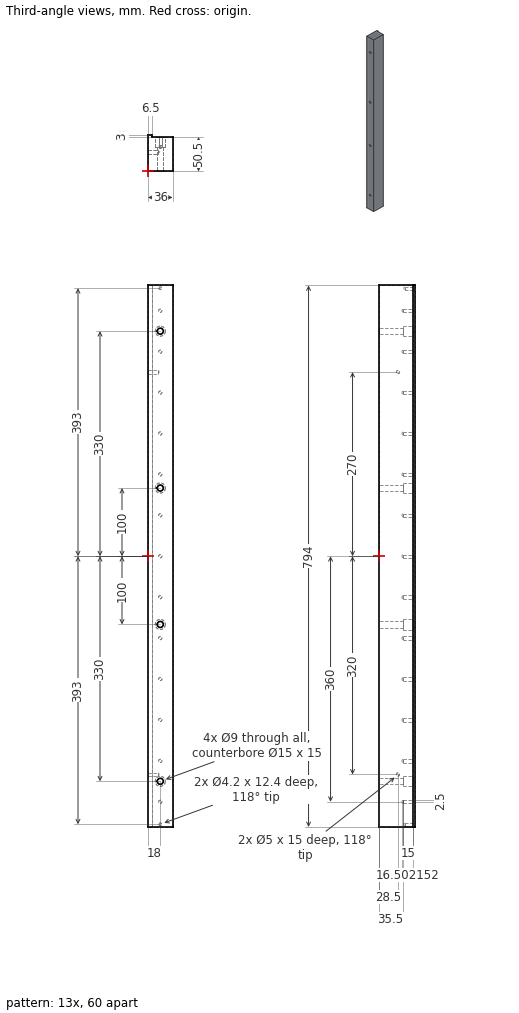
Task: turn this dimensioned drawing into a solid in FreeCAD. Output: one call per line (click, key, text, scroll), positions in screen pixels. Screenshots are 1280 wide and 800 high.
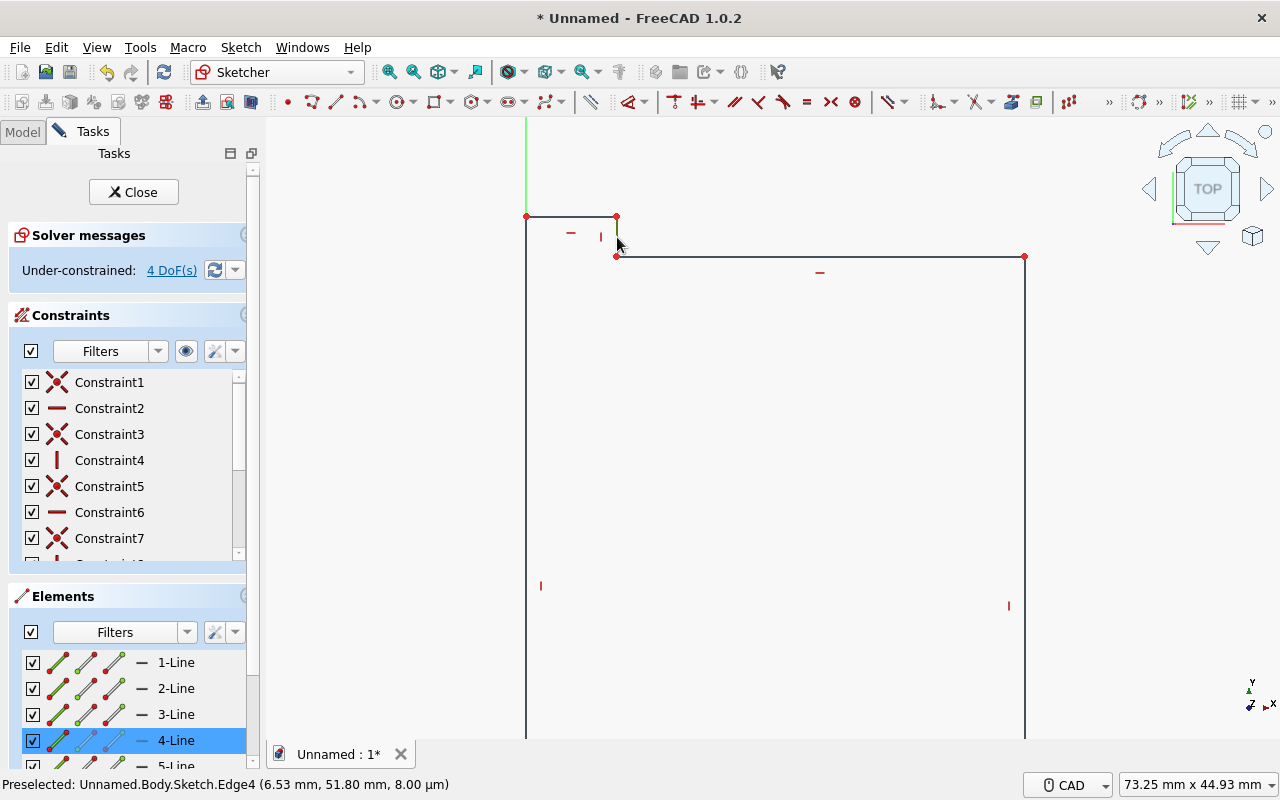
key(i)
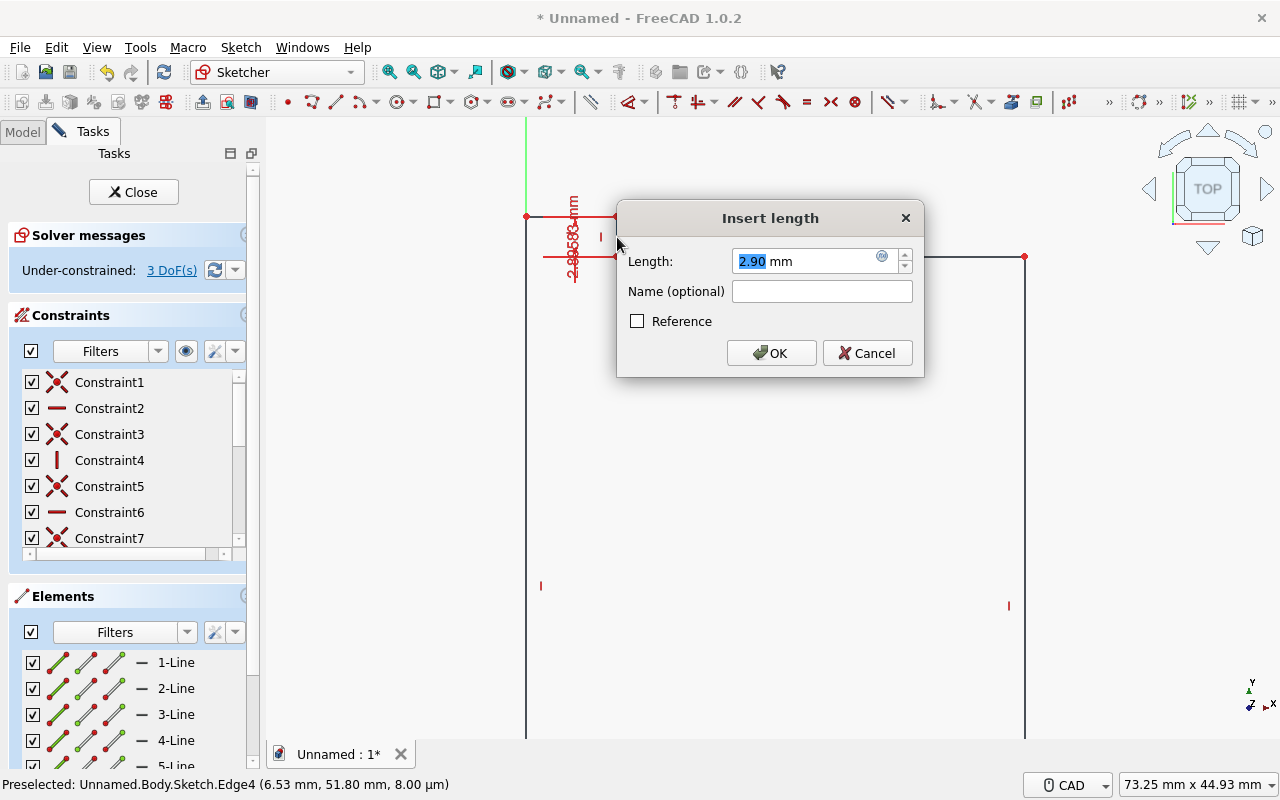
text(3)
key(Return)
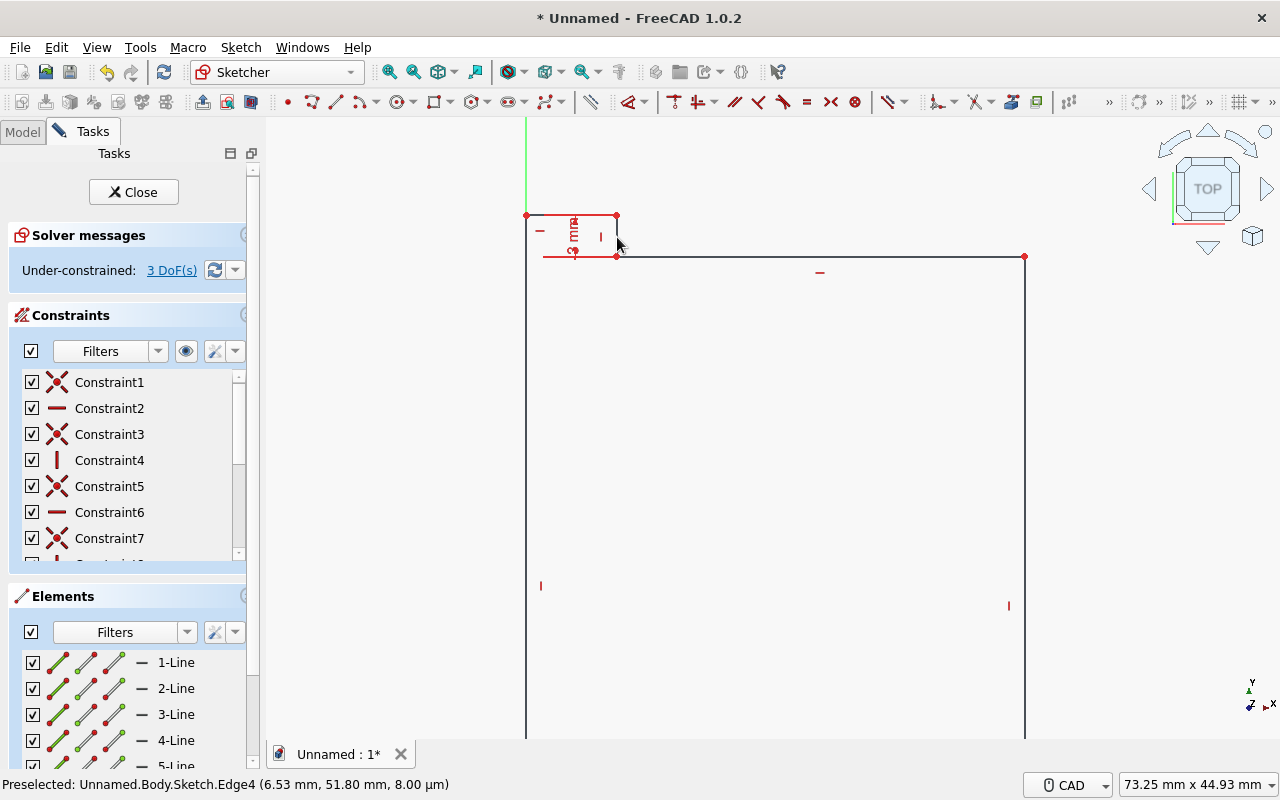
scroll(618, 237, down, 3)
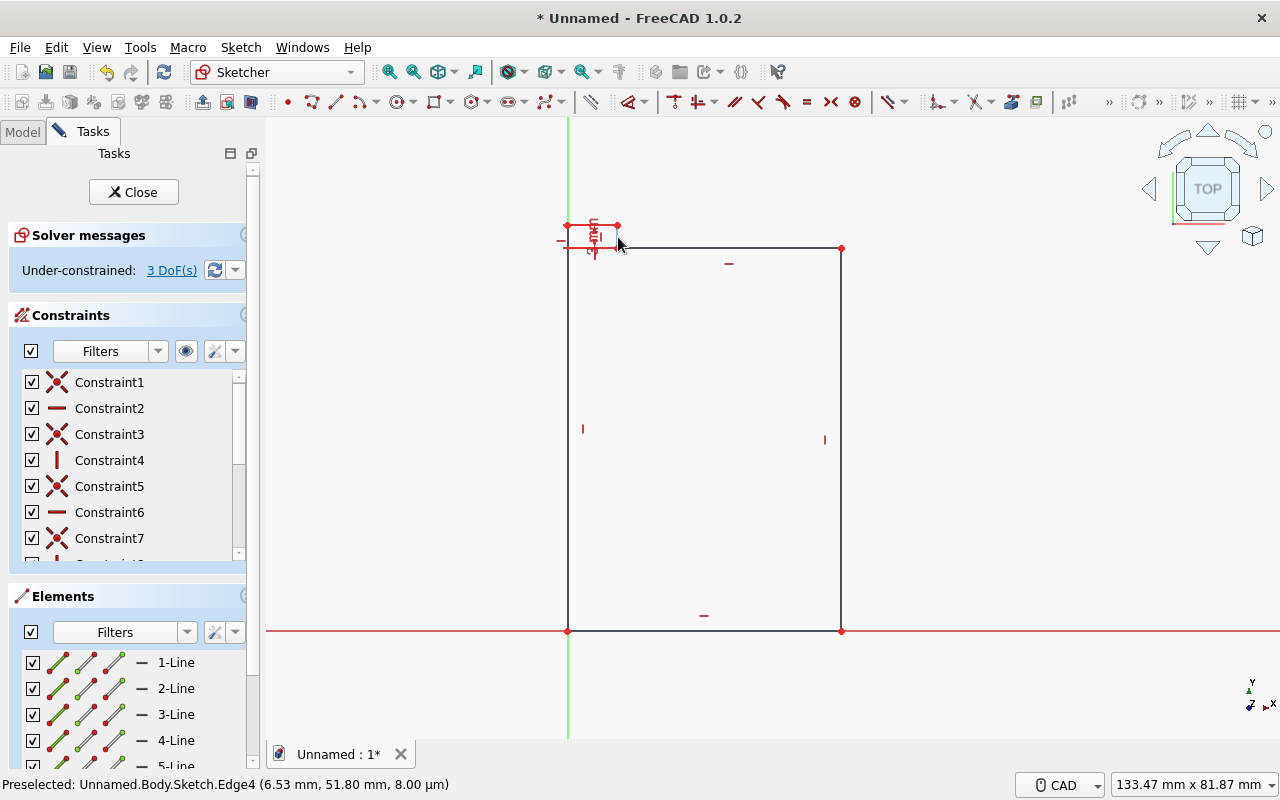
click(650, 631)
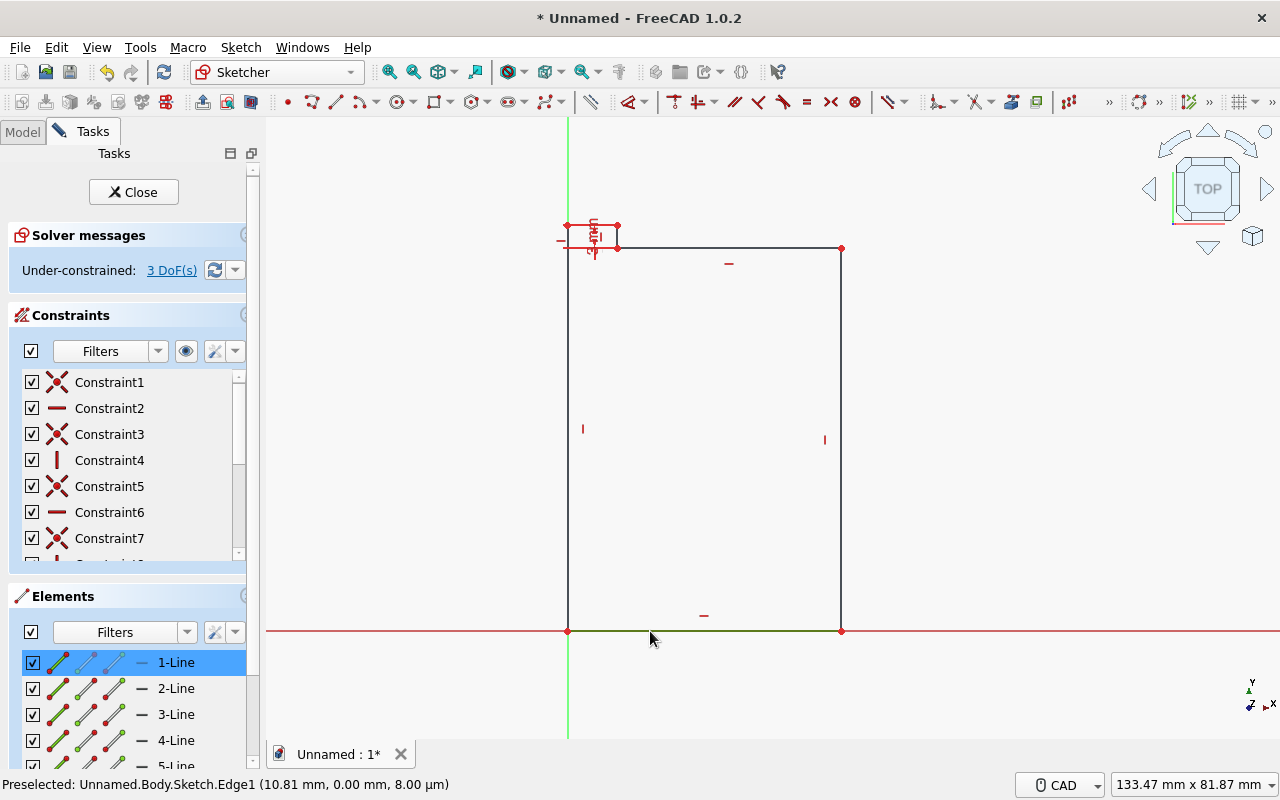
click(646, 102)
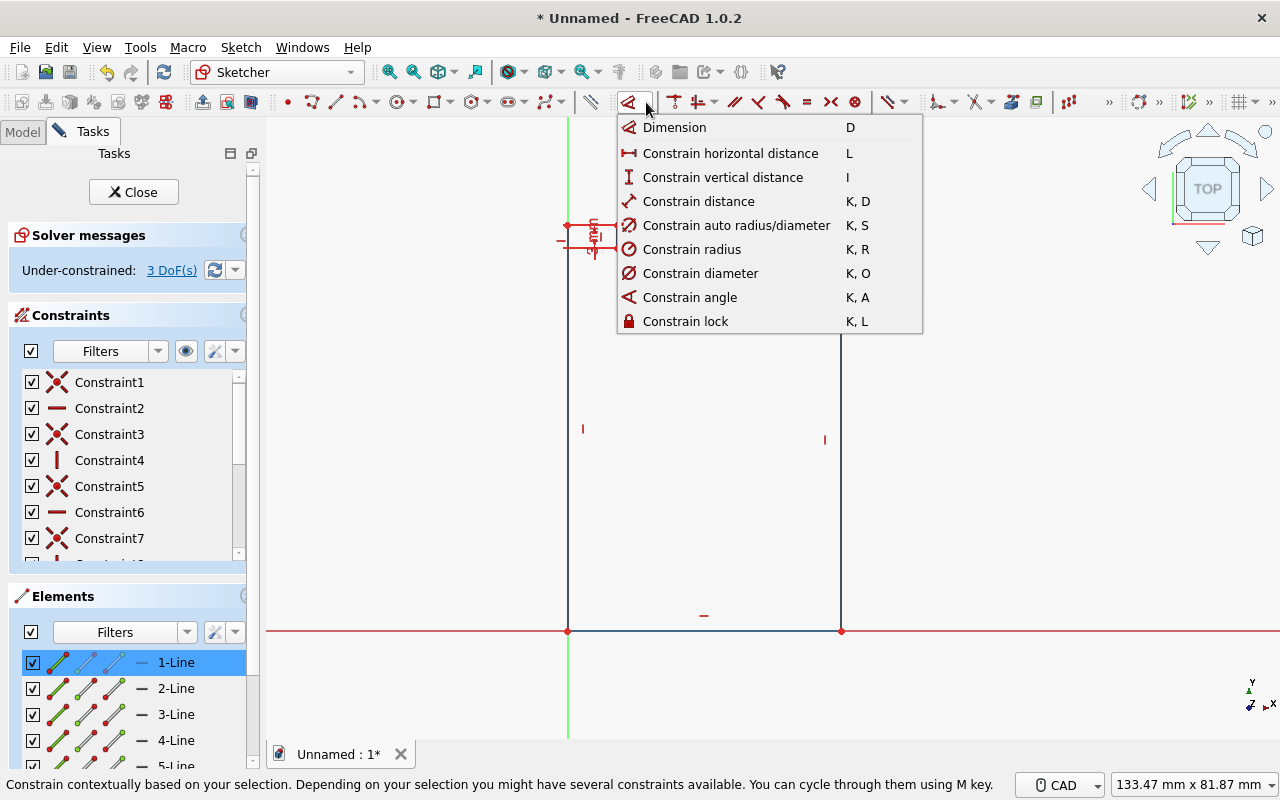
click(770, 153)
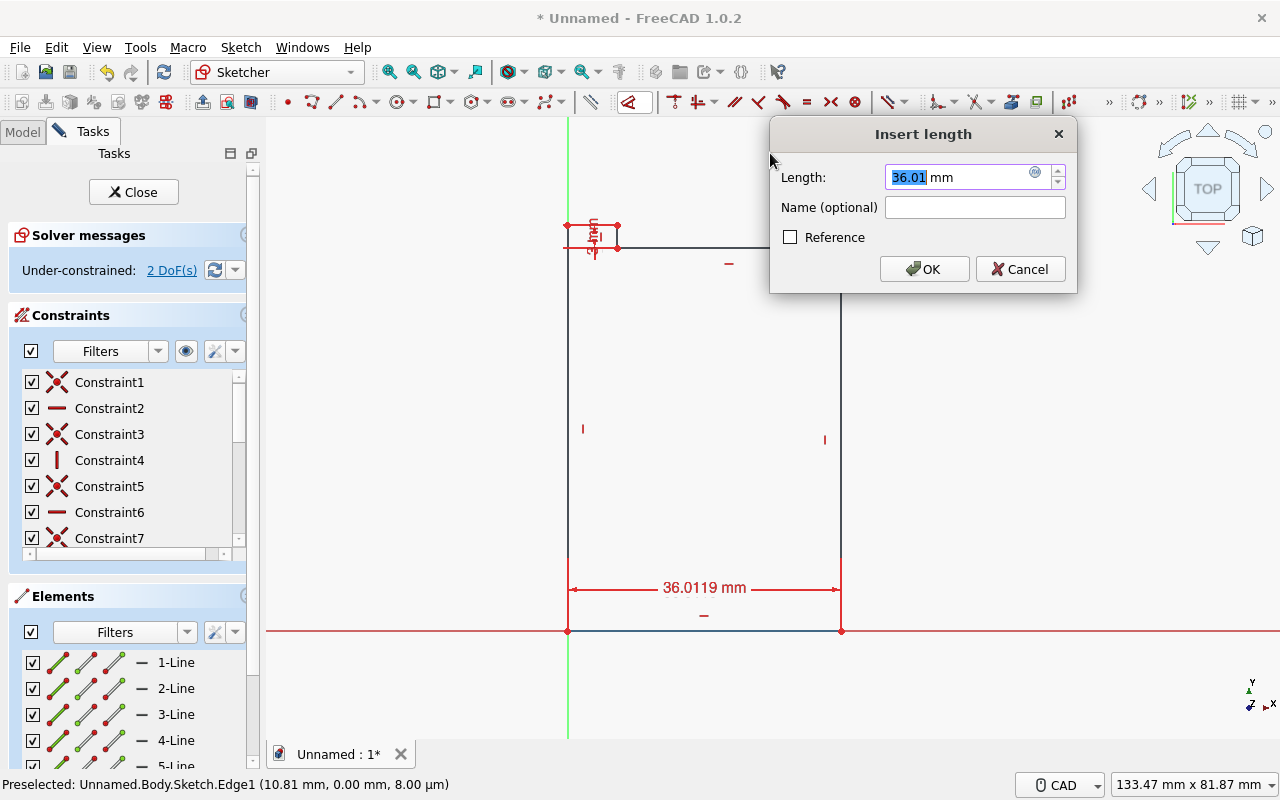
text(36)
key(Return)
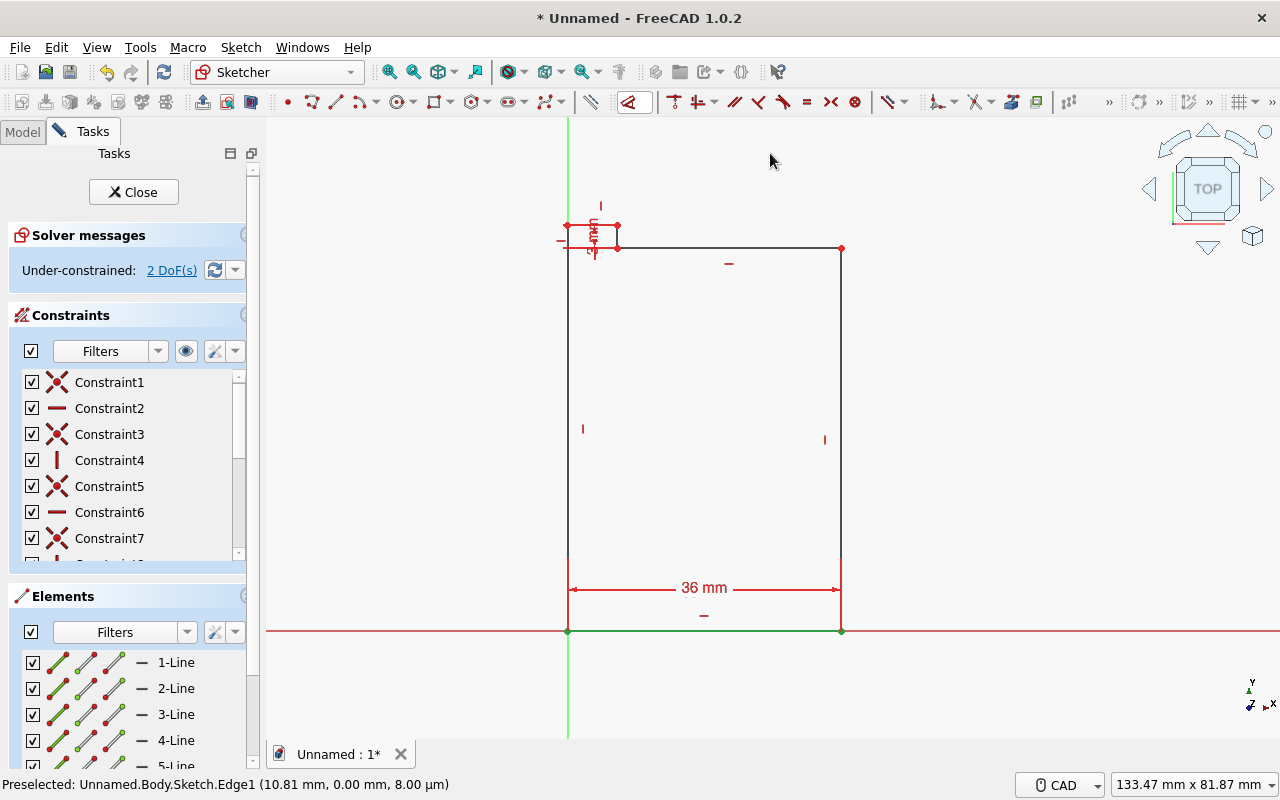
click(603, 225)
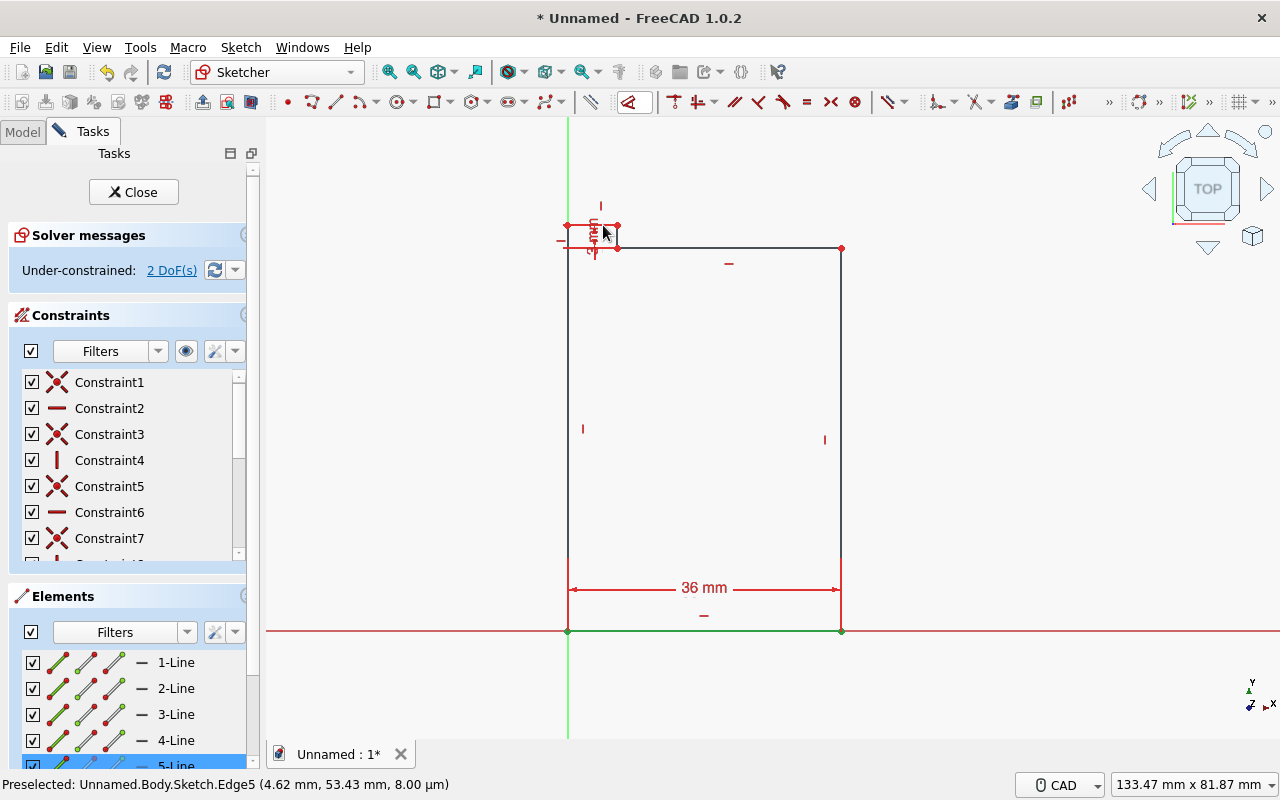
click(646, 102)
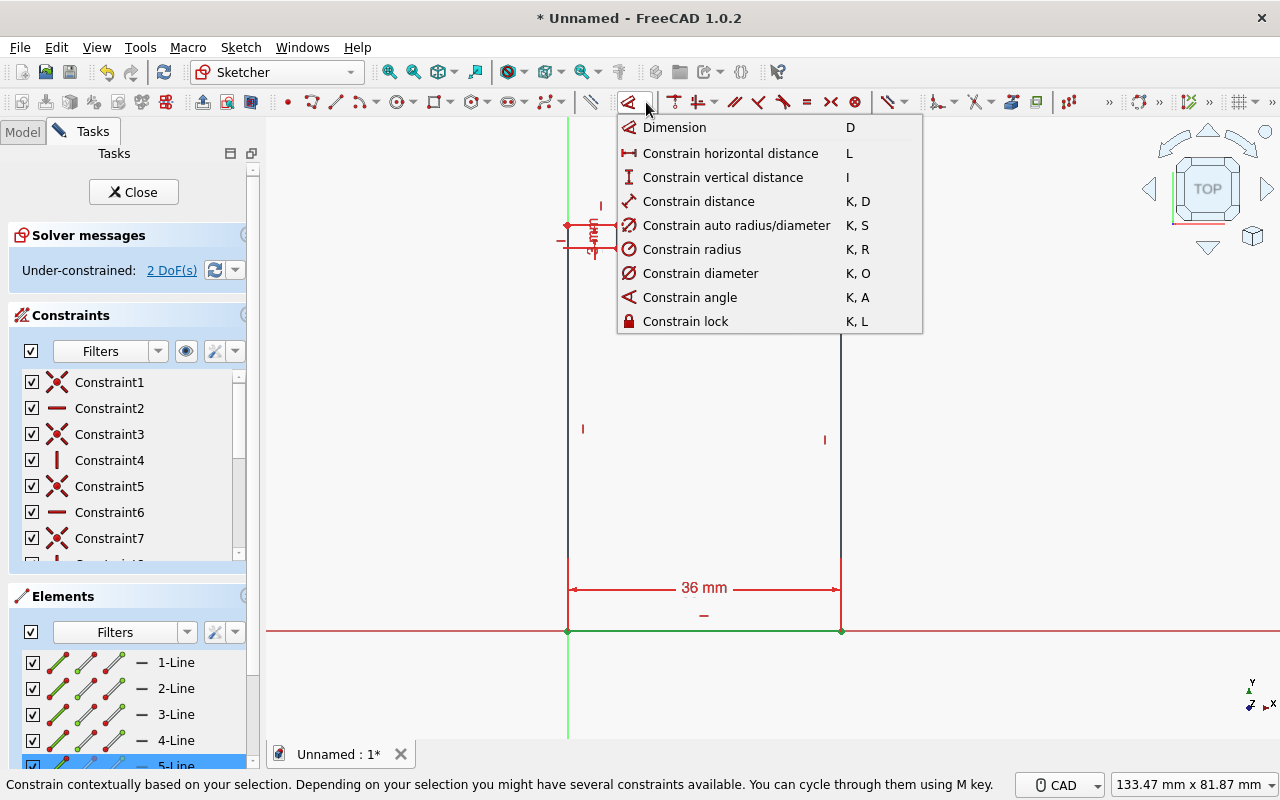
click(770, 153)